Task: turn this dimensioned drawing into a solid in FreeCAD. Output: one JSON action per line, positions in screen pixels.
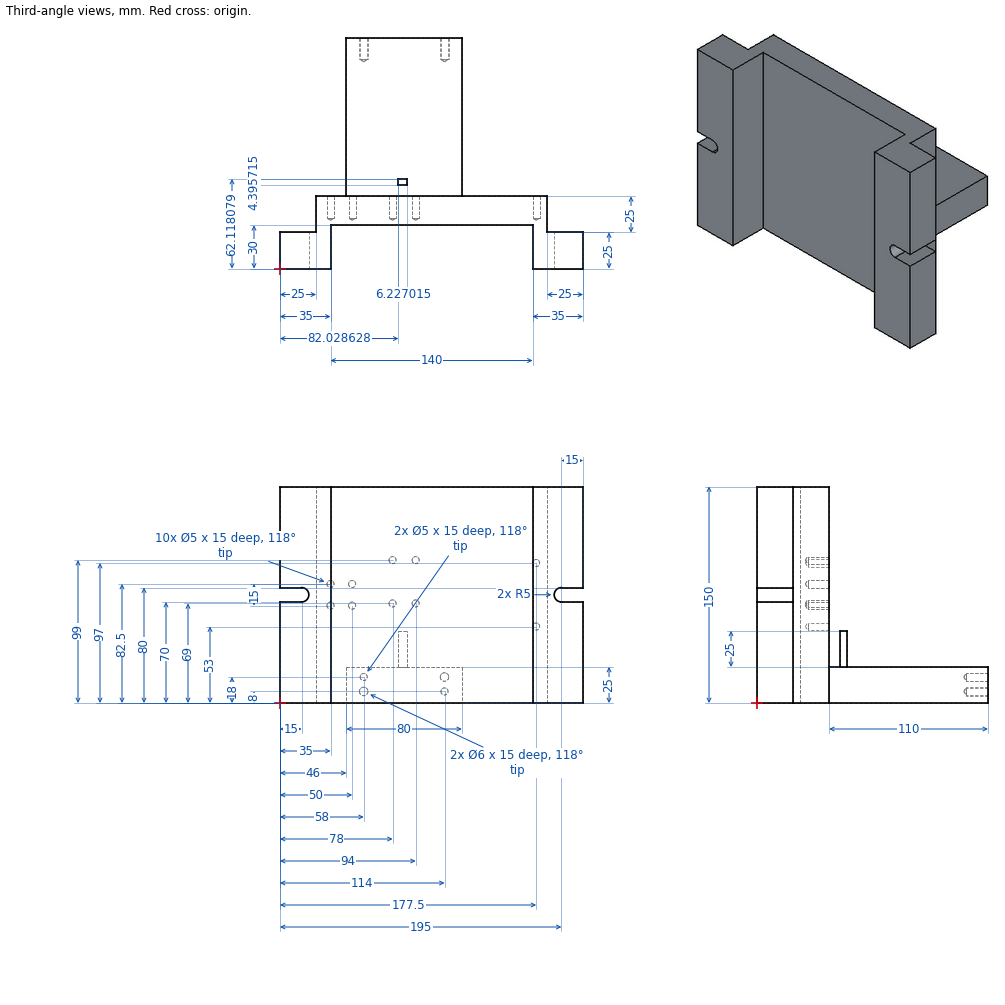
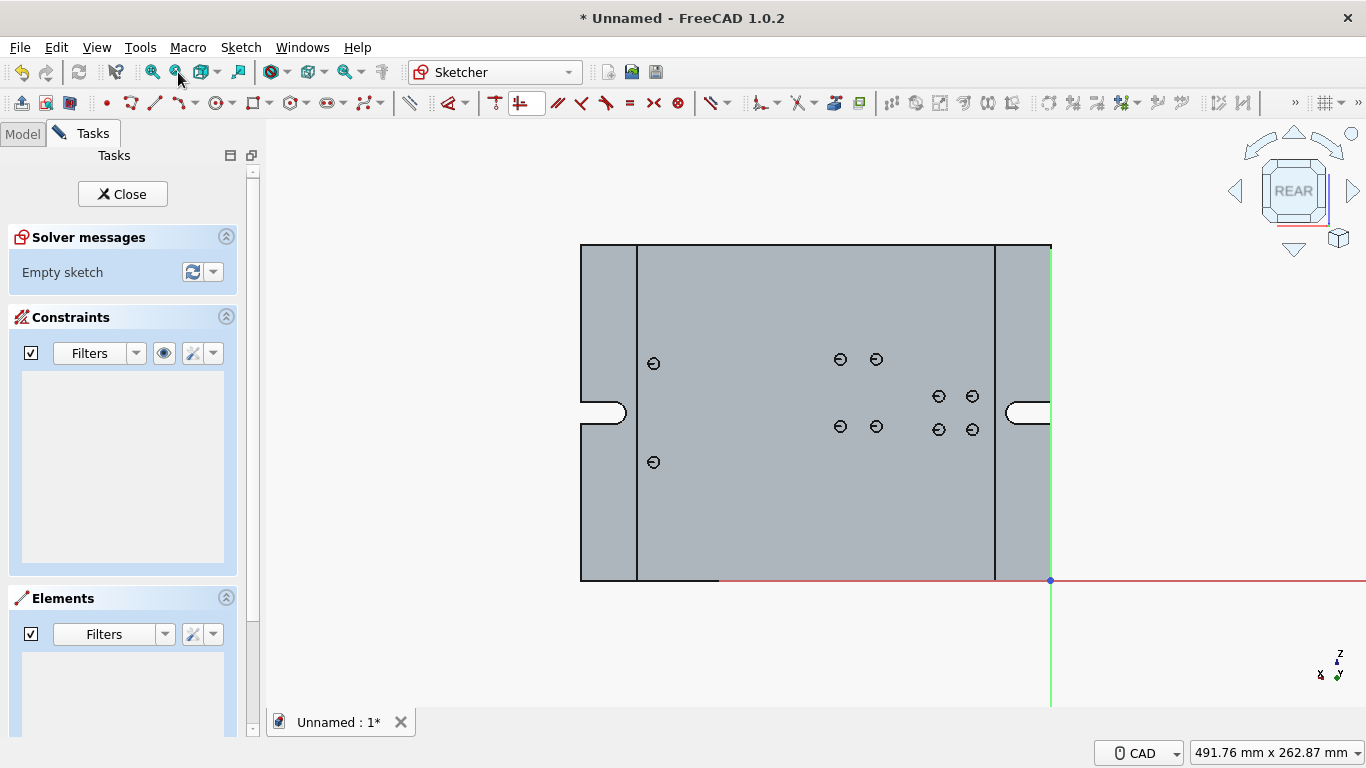
{"action": "scroll", "coordinate": [1043, 667], "scroll_direction": "up", "scroll_amount": 4}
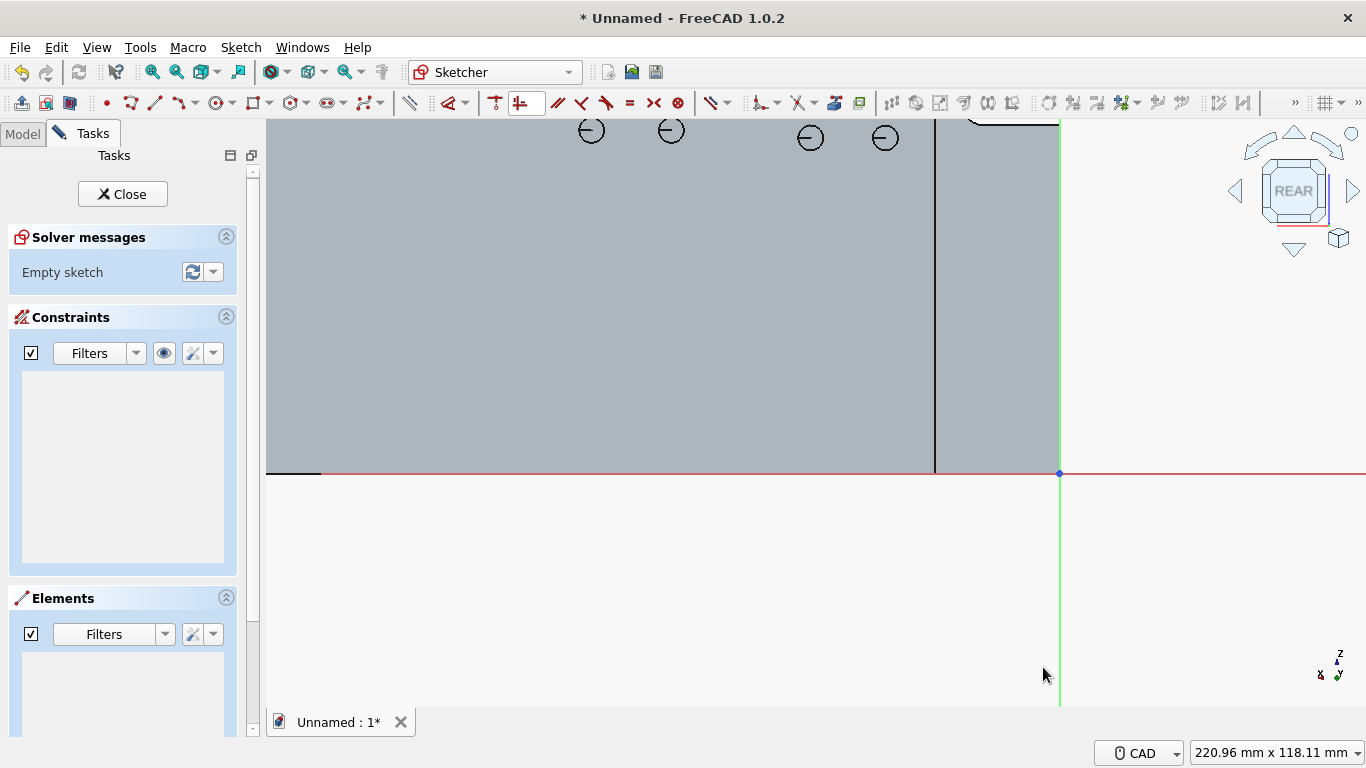
{"action": "left_click", "coordinate": [254, 104]}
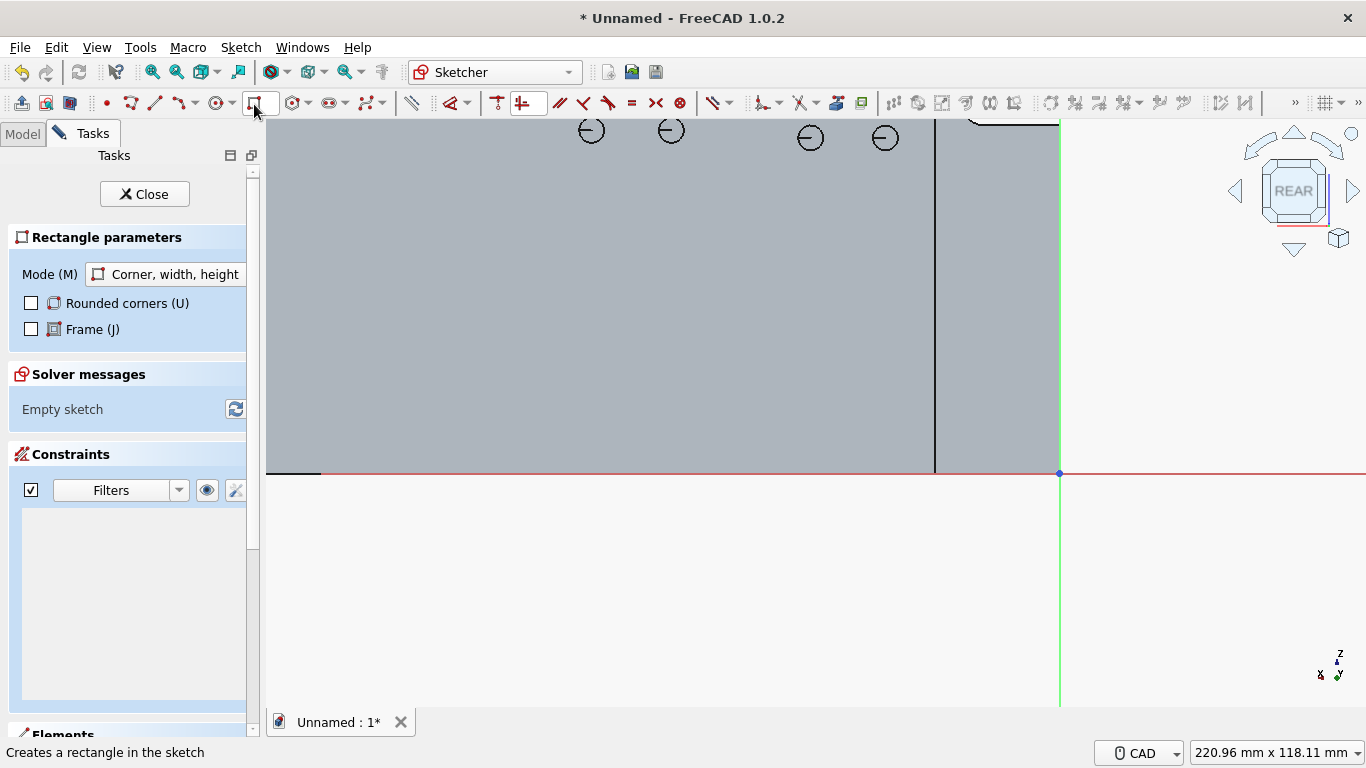
{"action": "left_click", "coordinate": [432, 349]}
{"action": "left_click", "coordinate": [831, 474]}
{"action": "key", "text": "Escape"}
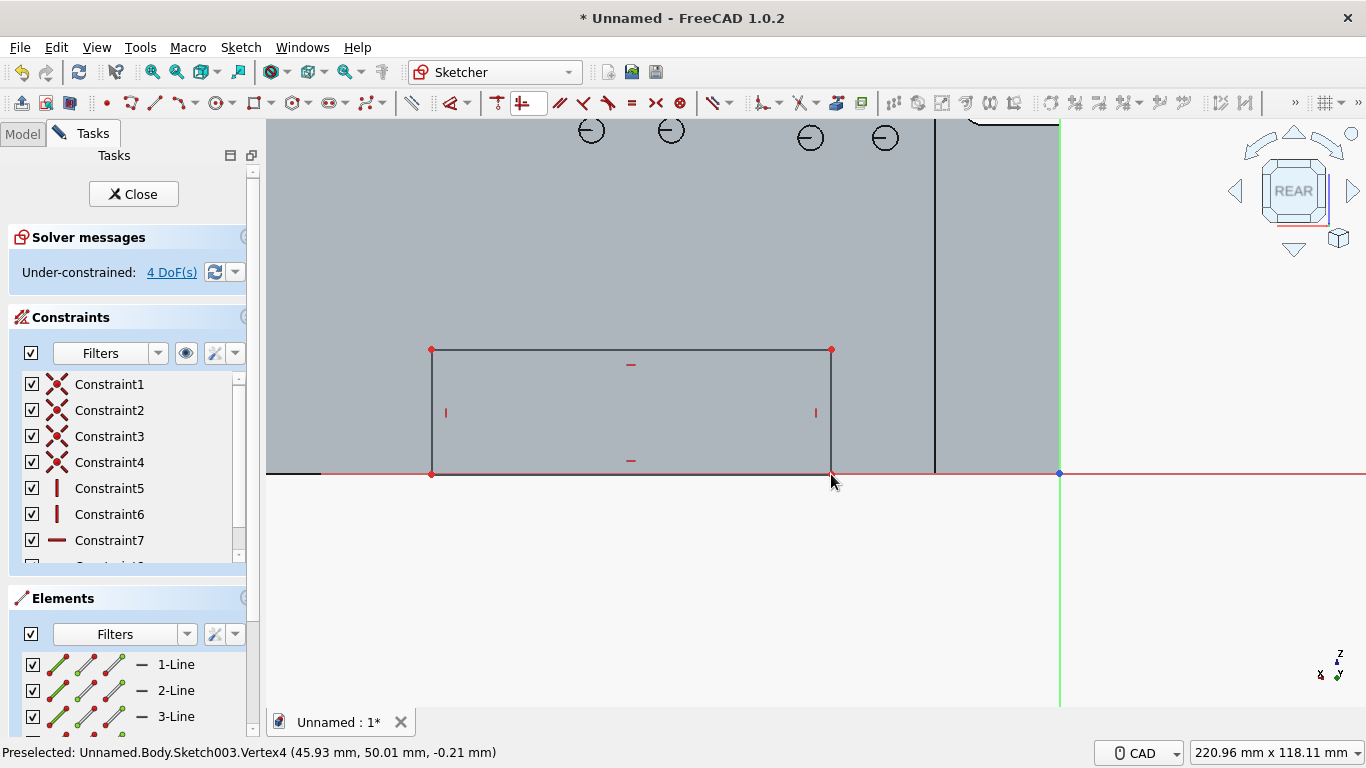
{"action": "left_click", "coordinate": [432, 475]}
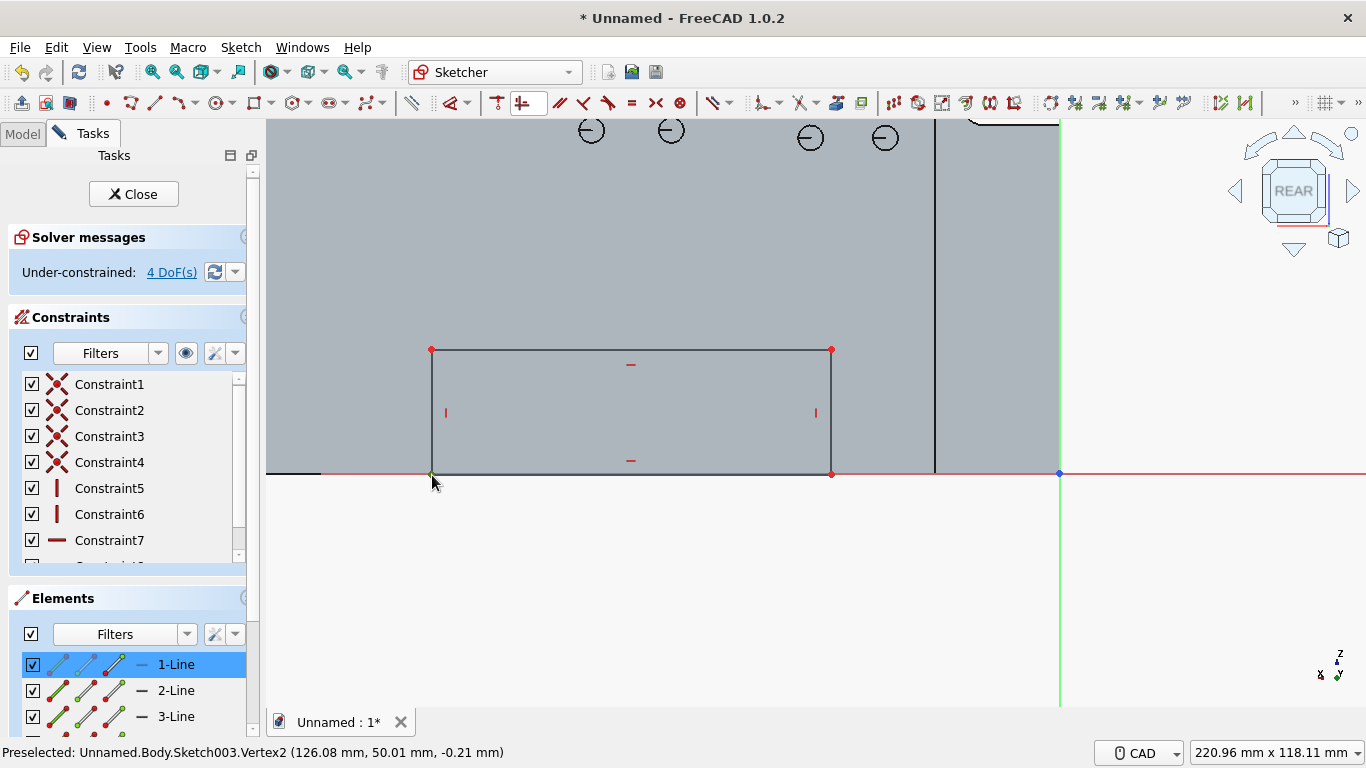
{"action": "left_click", "coordinate": [359, 474]}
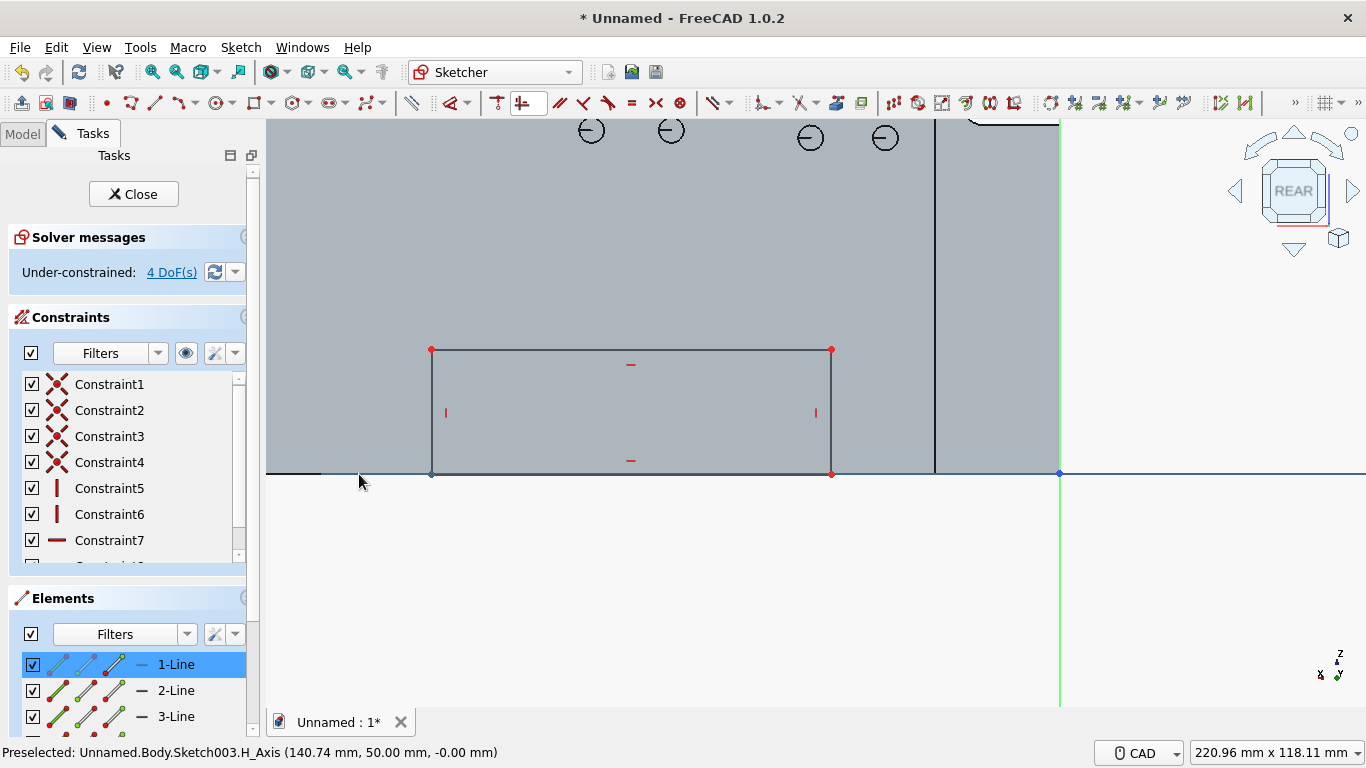
{"action": "left_click", "coordinate": [498, 104]}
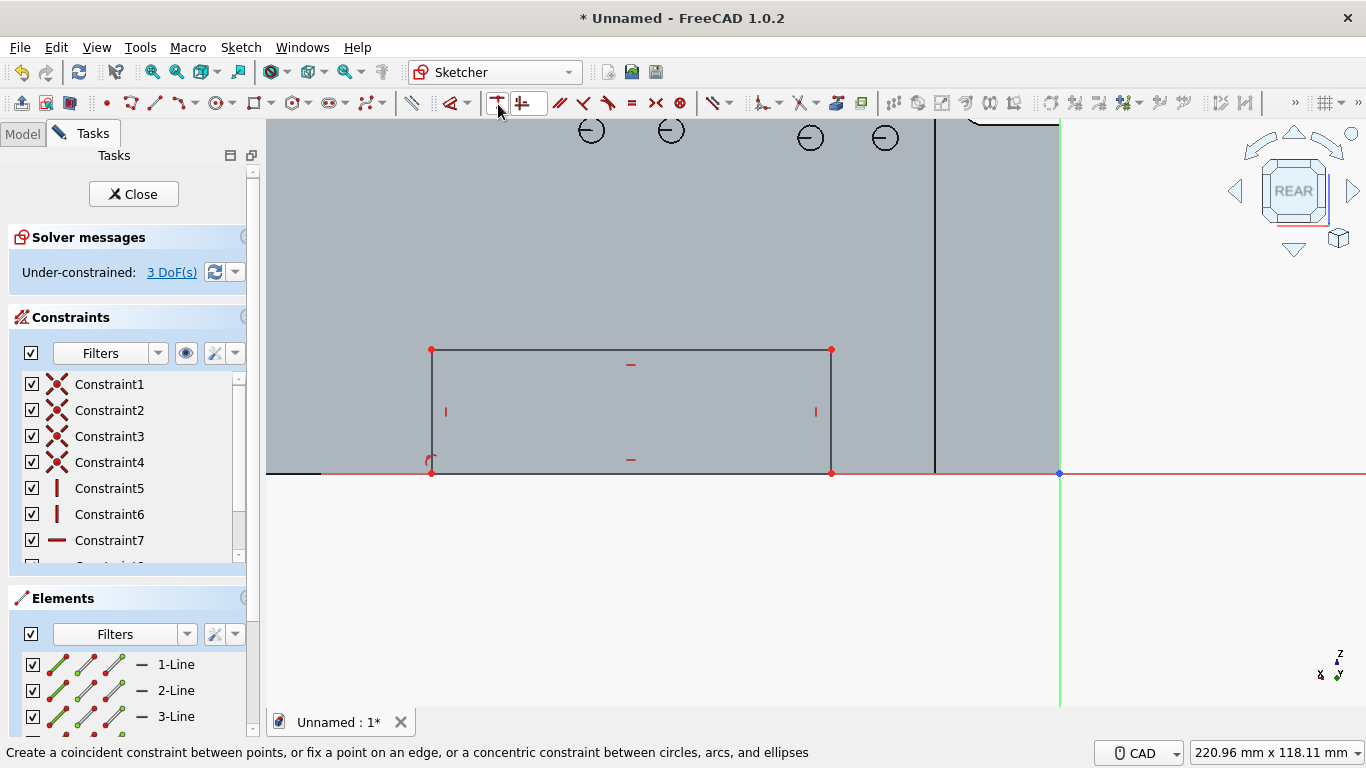
{"action": "left_click", "coordinate": [450, 104]}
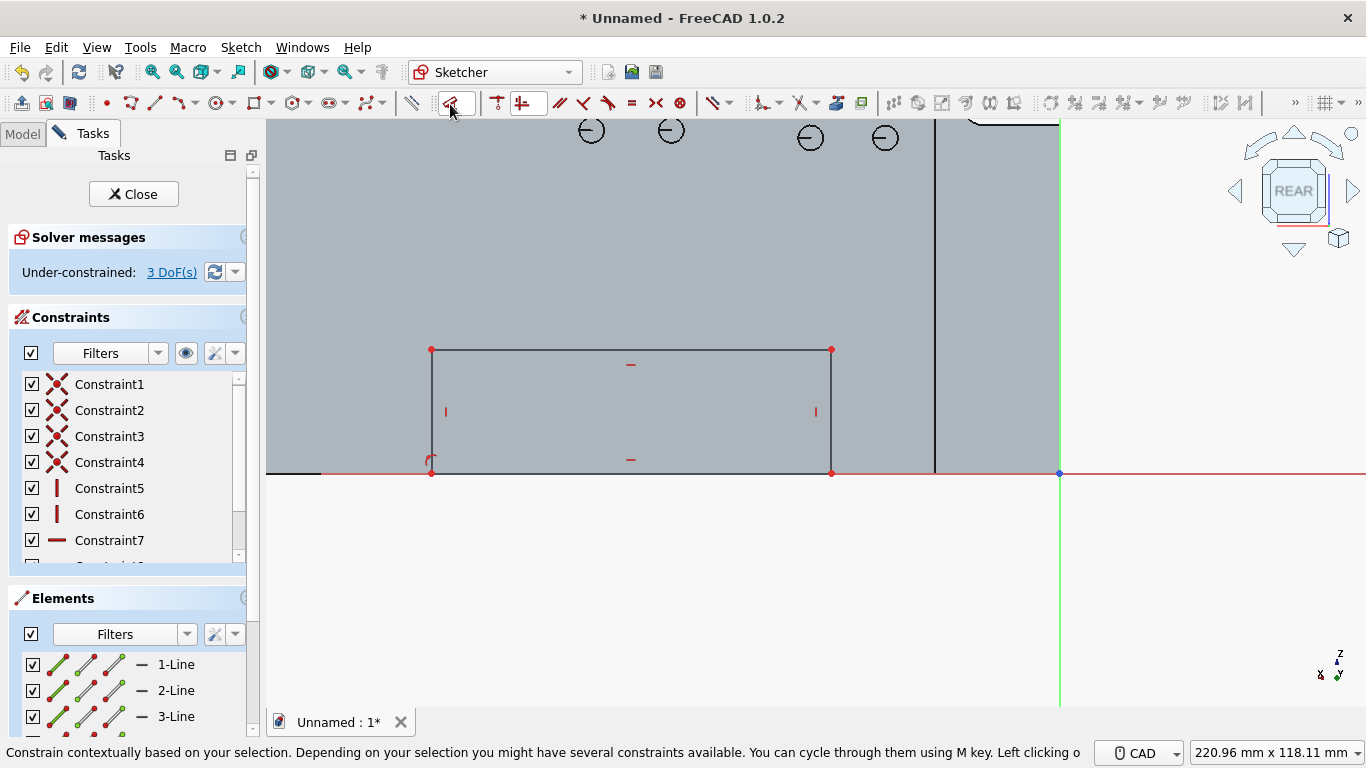
{"action": "left_click", "coordinate": [432, 387]}
{"action": "left_click", "coordinate": [398, 412]}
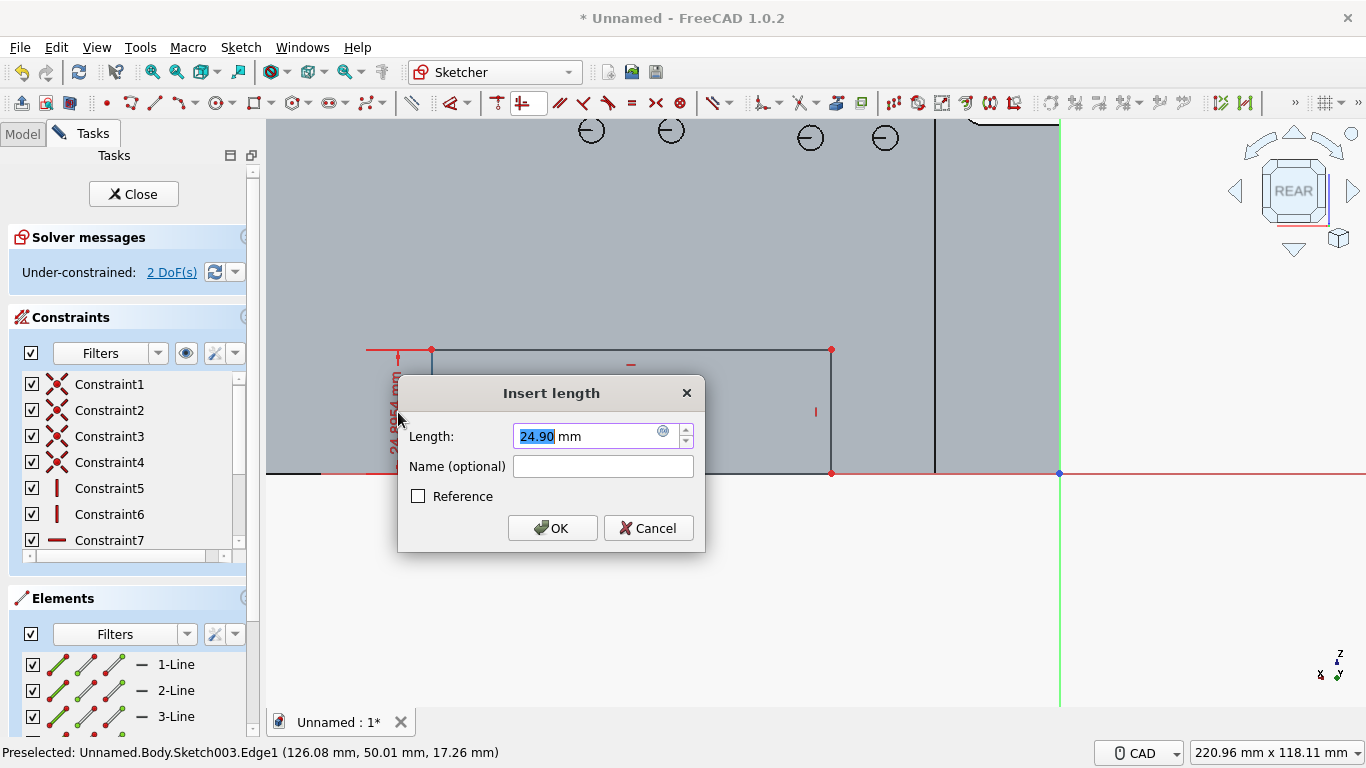
{"action": "type", "text": "25"}
{"action": "key", "text": "Return"}